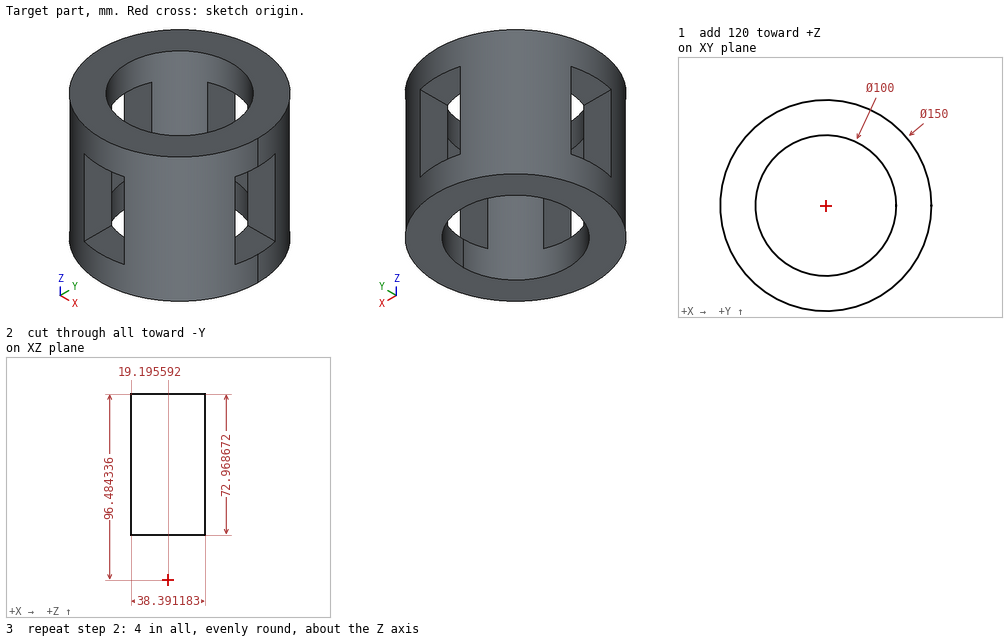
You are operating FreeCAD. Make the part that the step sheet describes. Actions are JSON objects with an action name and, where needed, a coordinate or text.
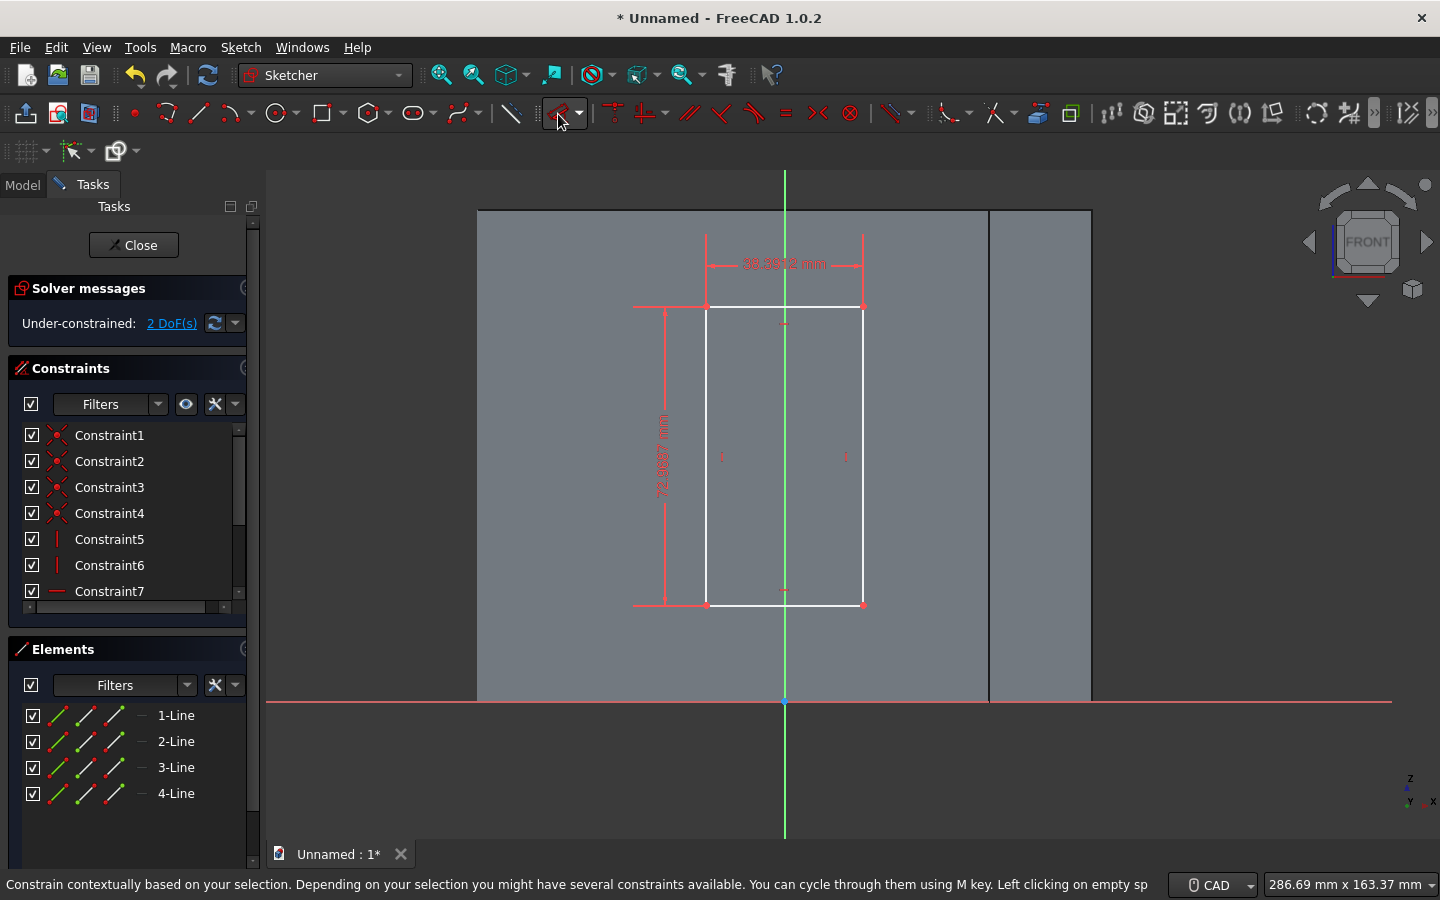
{"action": "left_click", "coordinate": [706, 307]}
{"action": "left_click", "coordinate": [745, 736]}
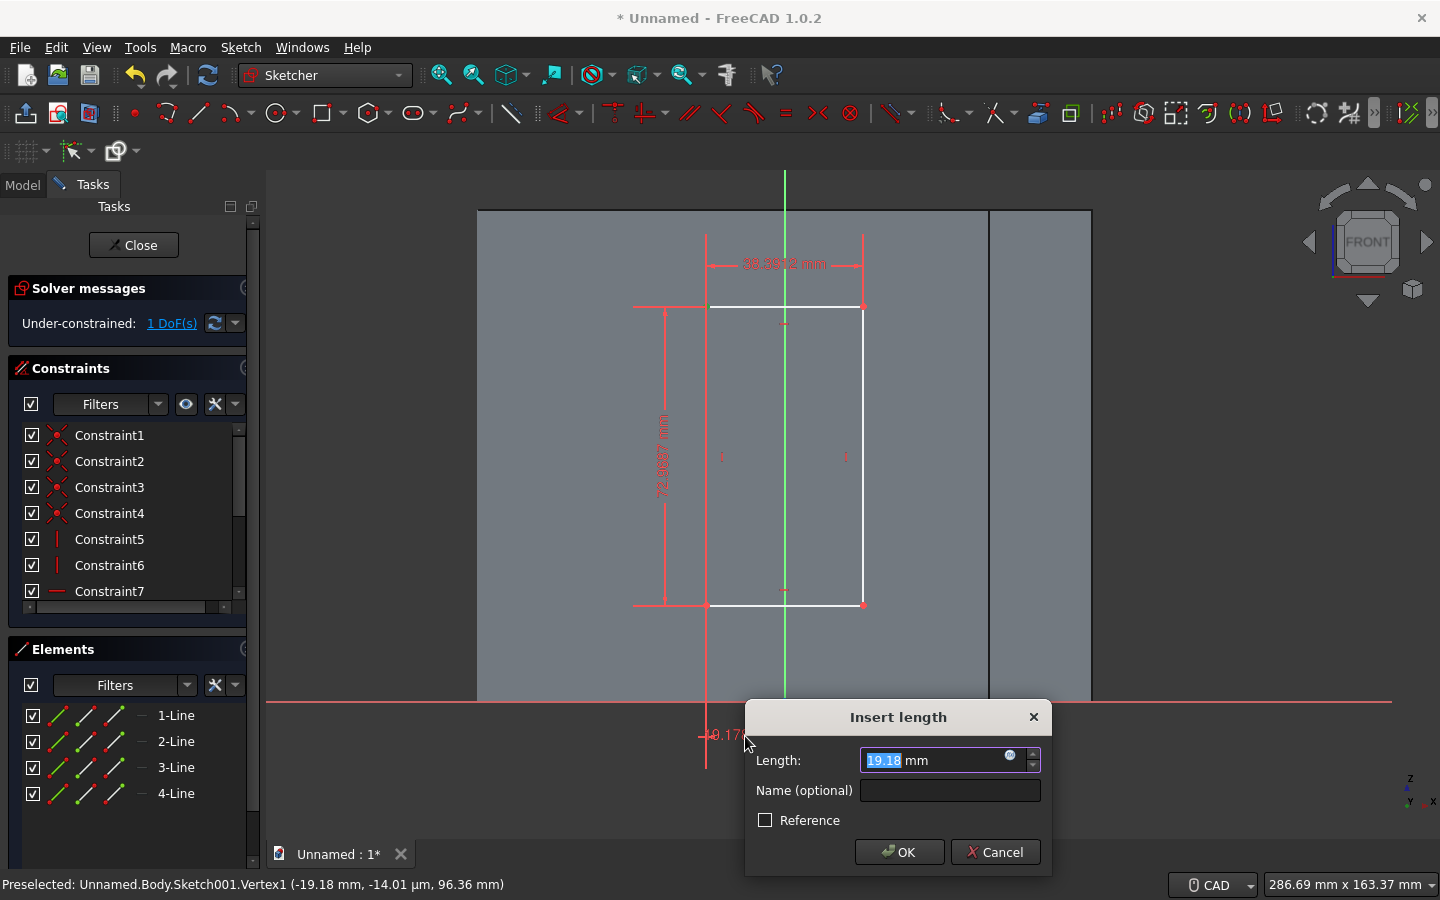
{"action": "type", "text": "19.195592"}
{"action": "key", "text": "Return"}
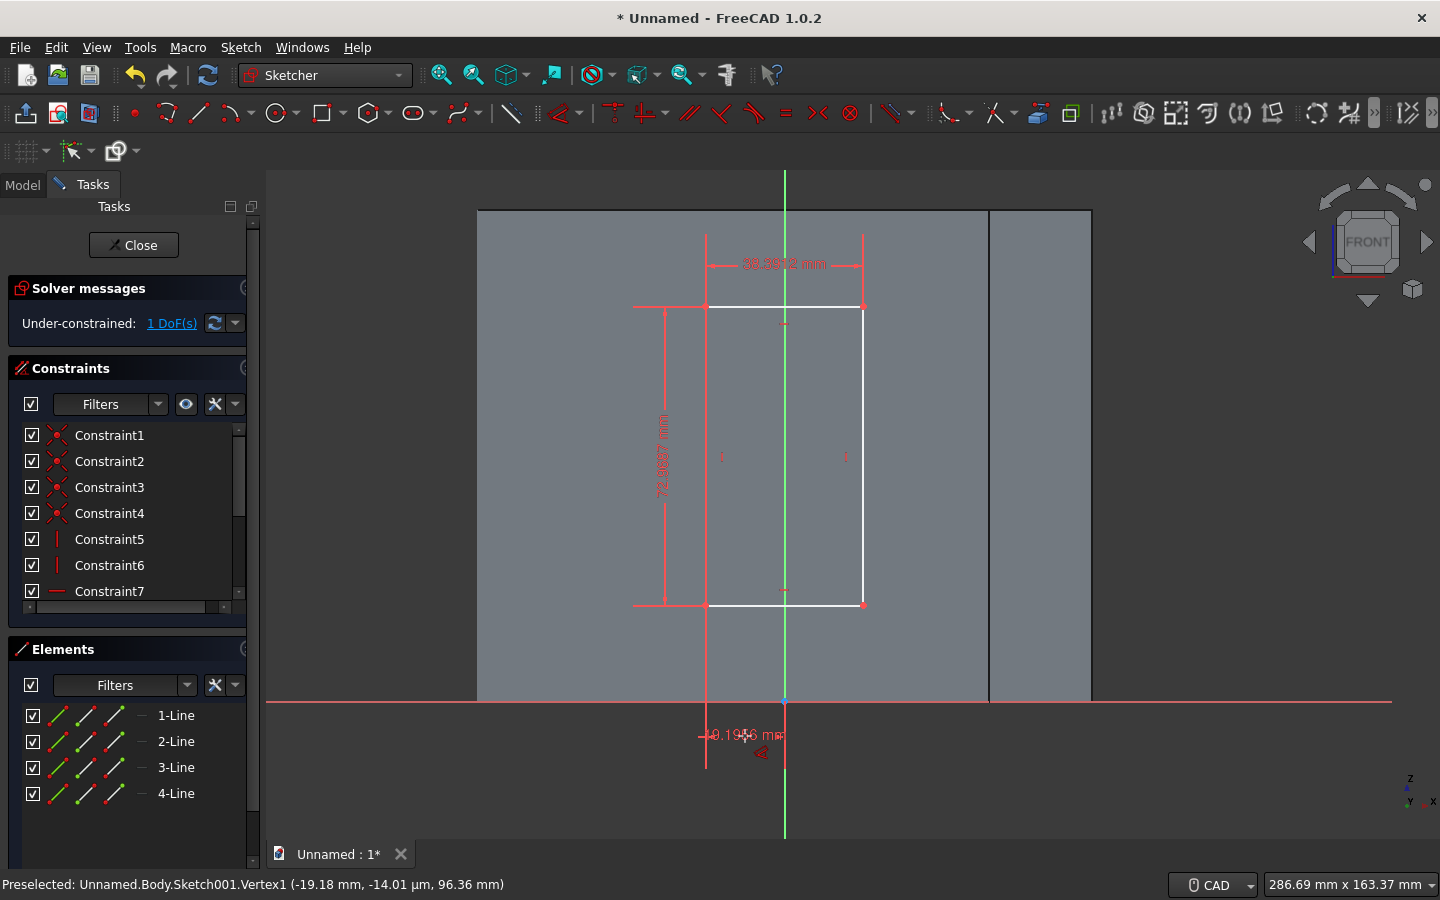
{"action": "left_click", "coordinate": [706, 307]}
{"action": "left_click", "coordinate": [672, 504]}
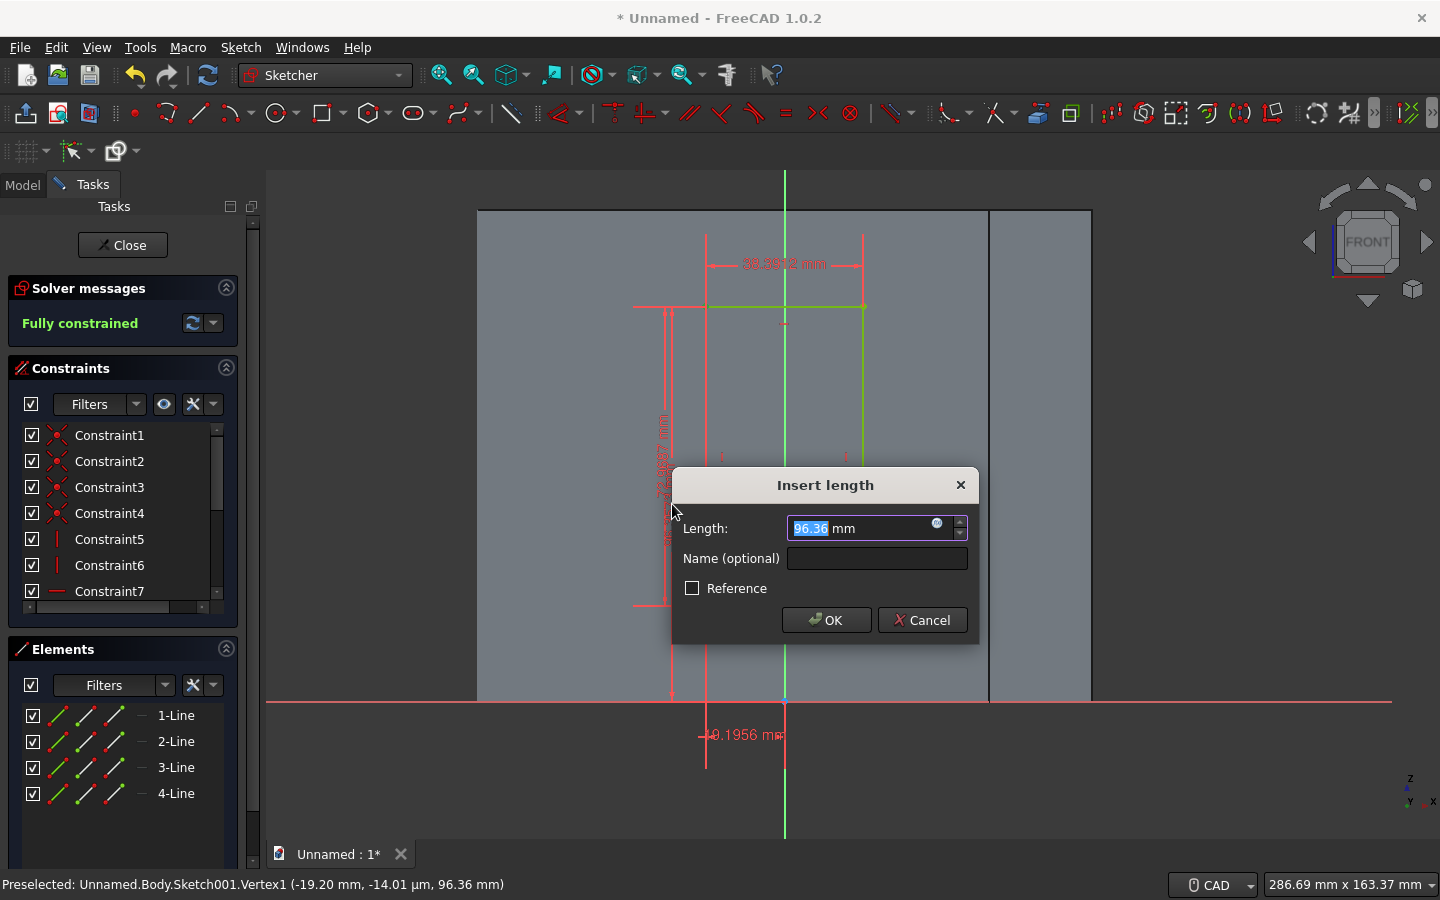
{"action": "type", "text": "96.484336"}
{"action": "key", "text": "Return"}
{"action": "key", "text": "Escape"}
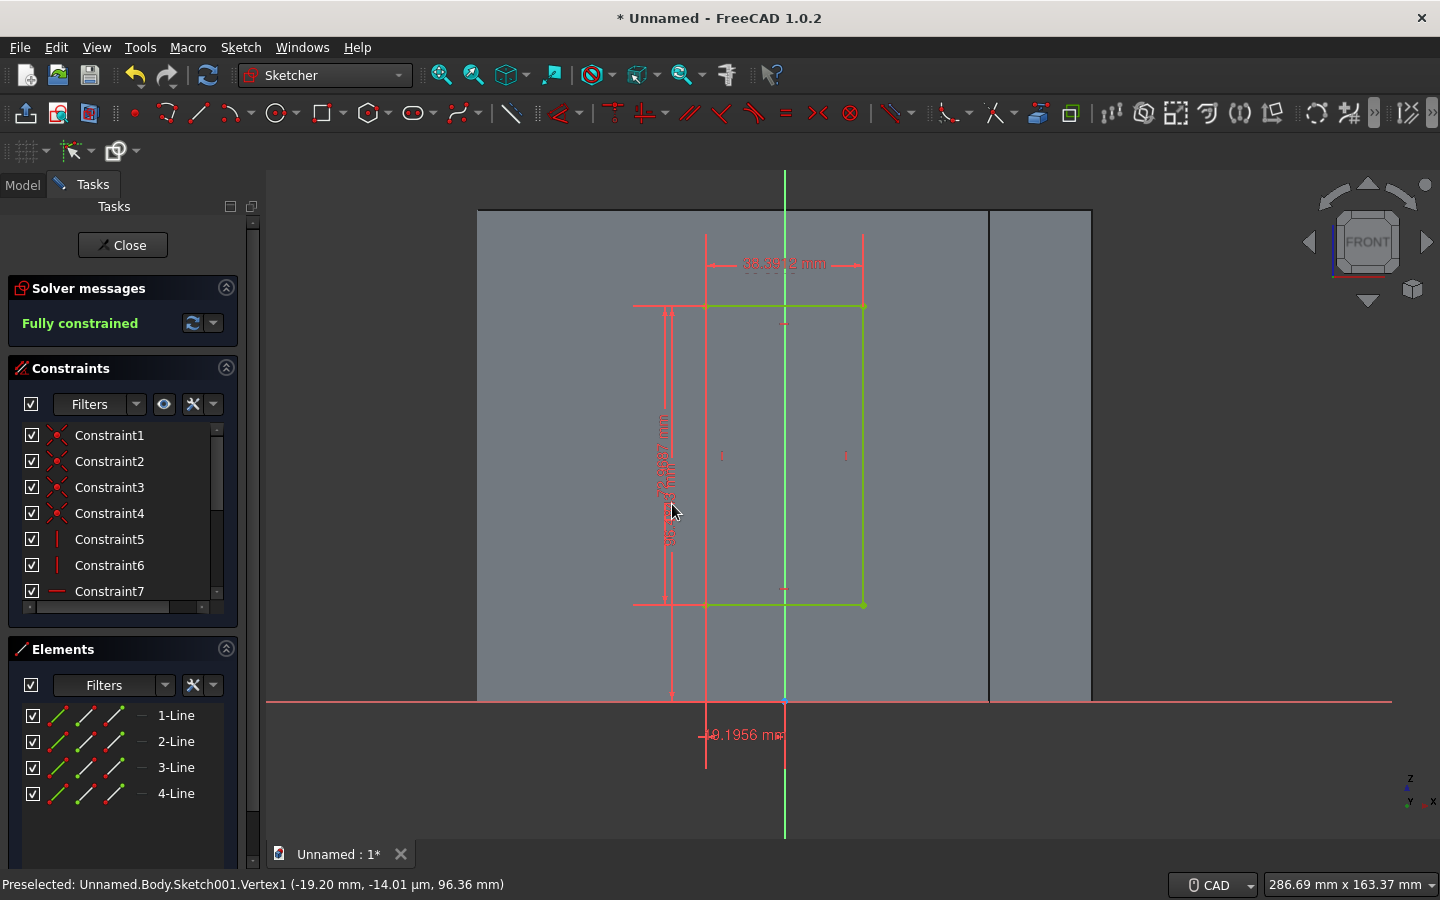
{"action": "left_click", "coordinate": [123, 245]}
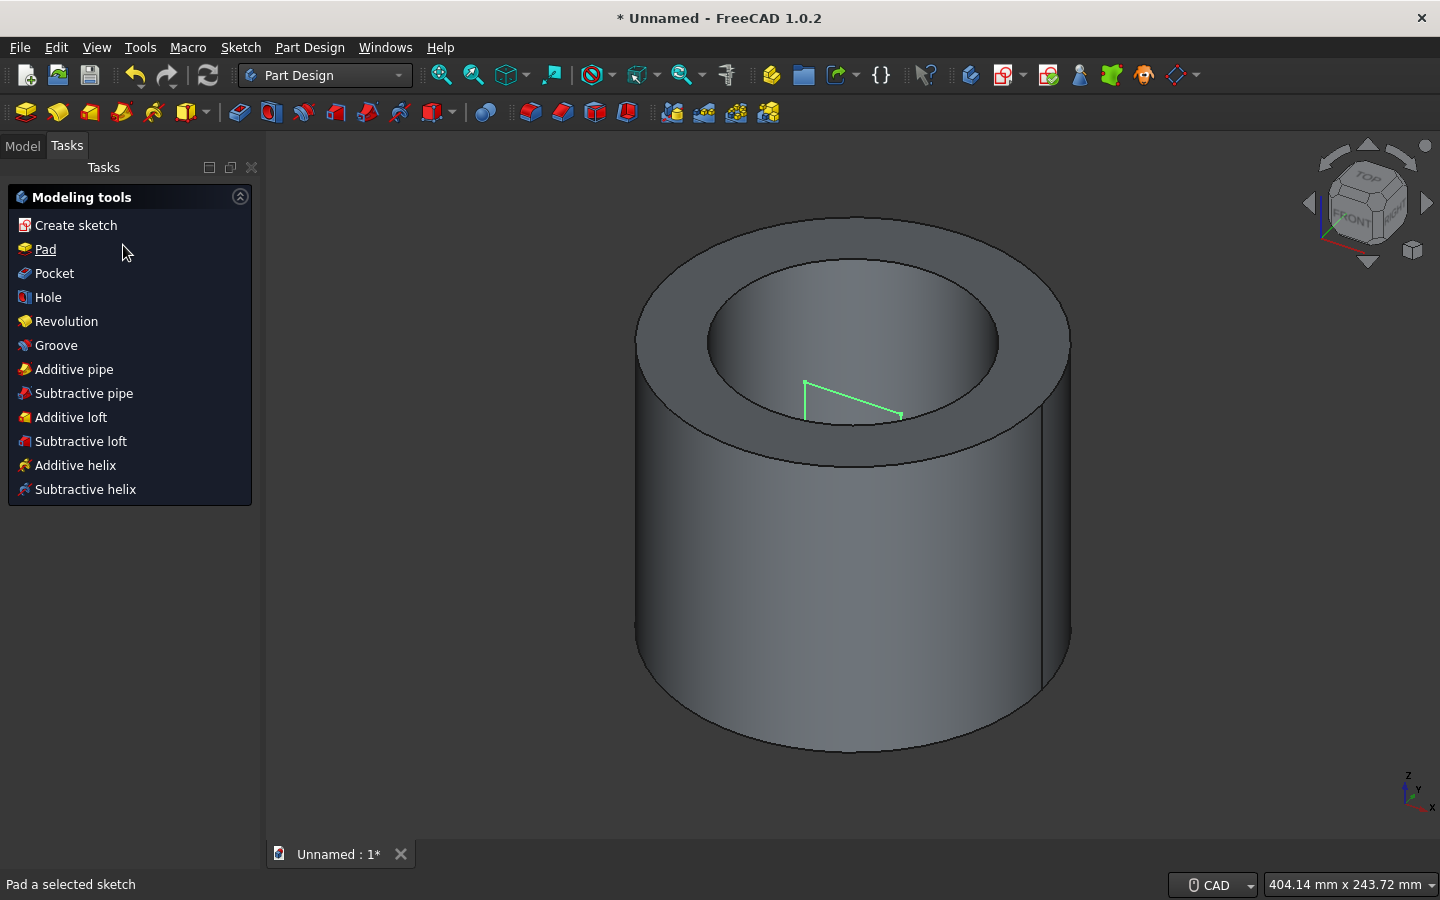
{"action": "left_click", "coordinate": [240, 112]}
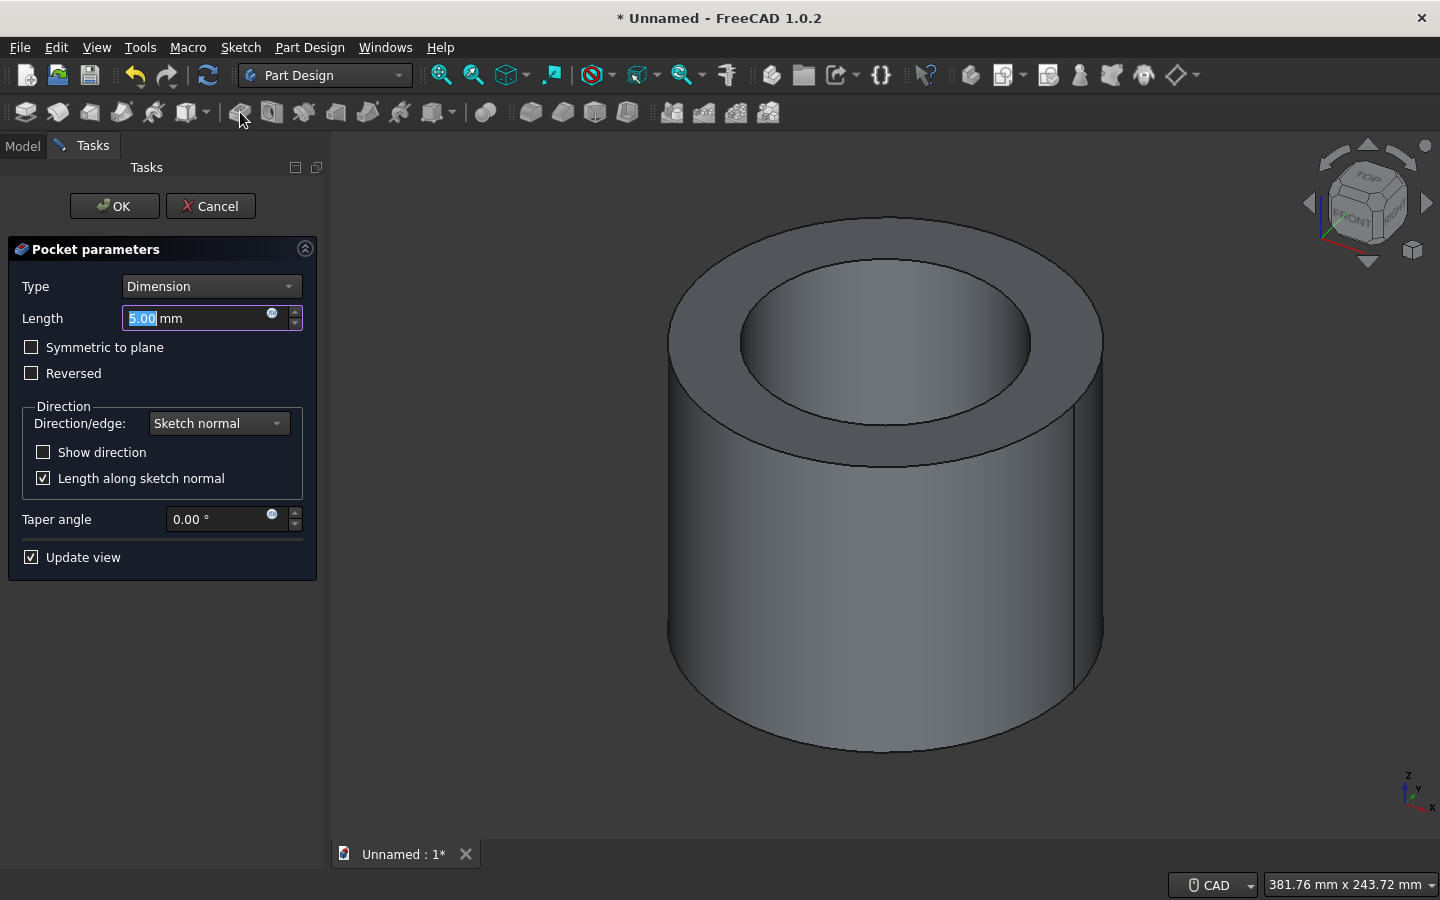
{"action": "left_click", "coordinate": [212, 286]}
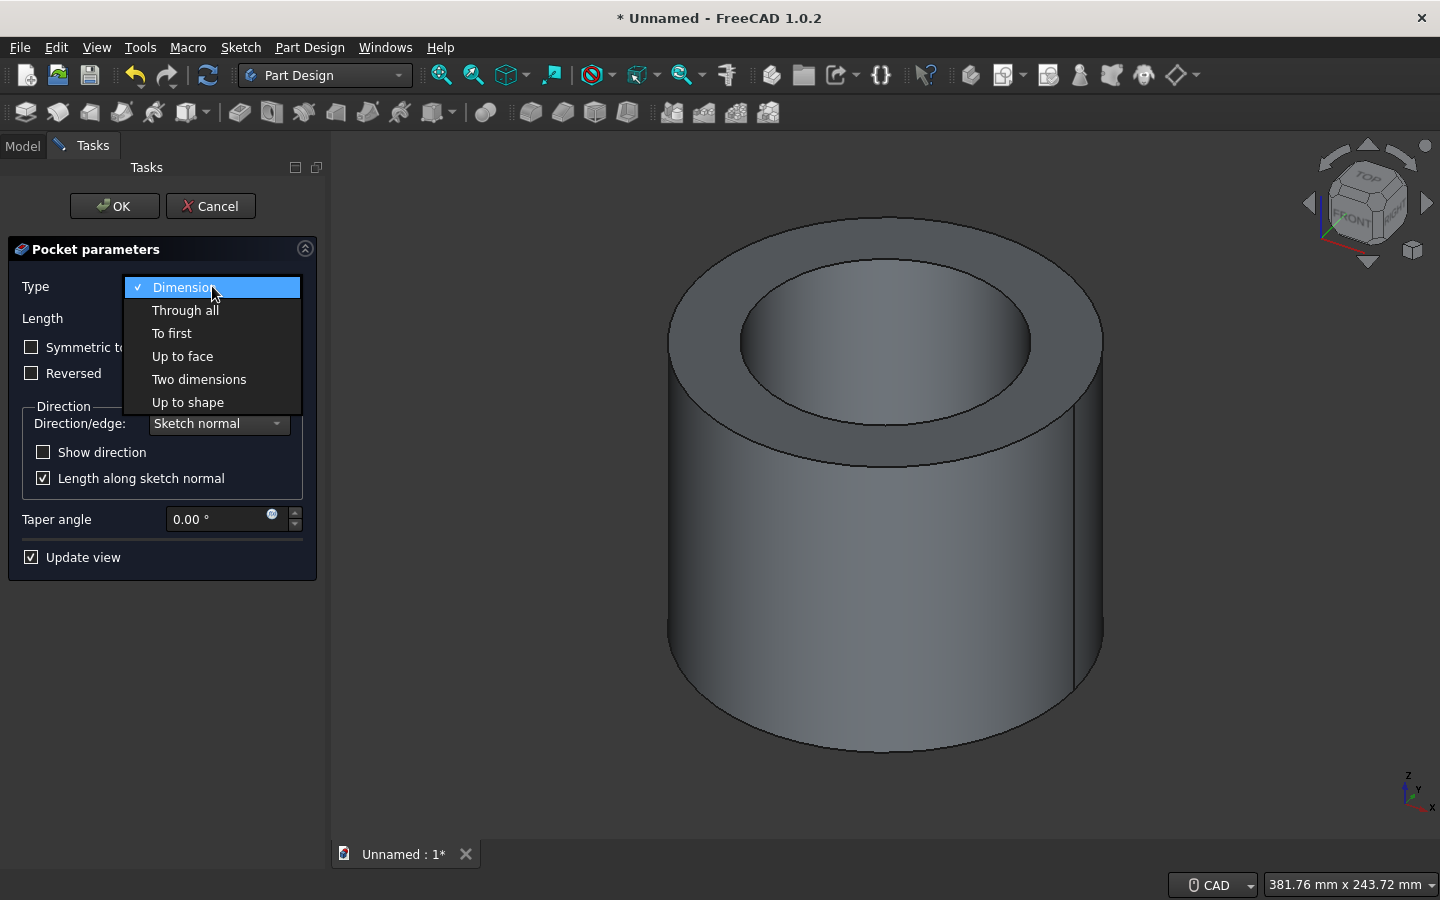
{"action": "left_click", "coordinate": [212, 310]}